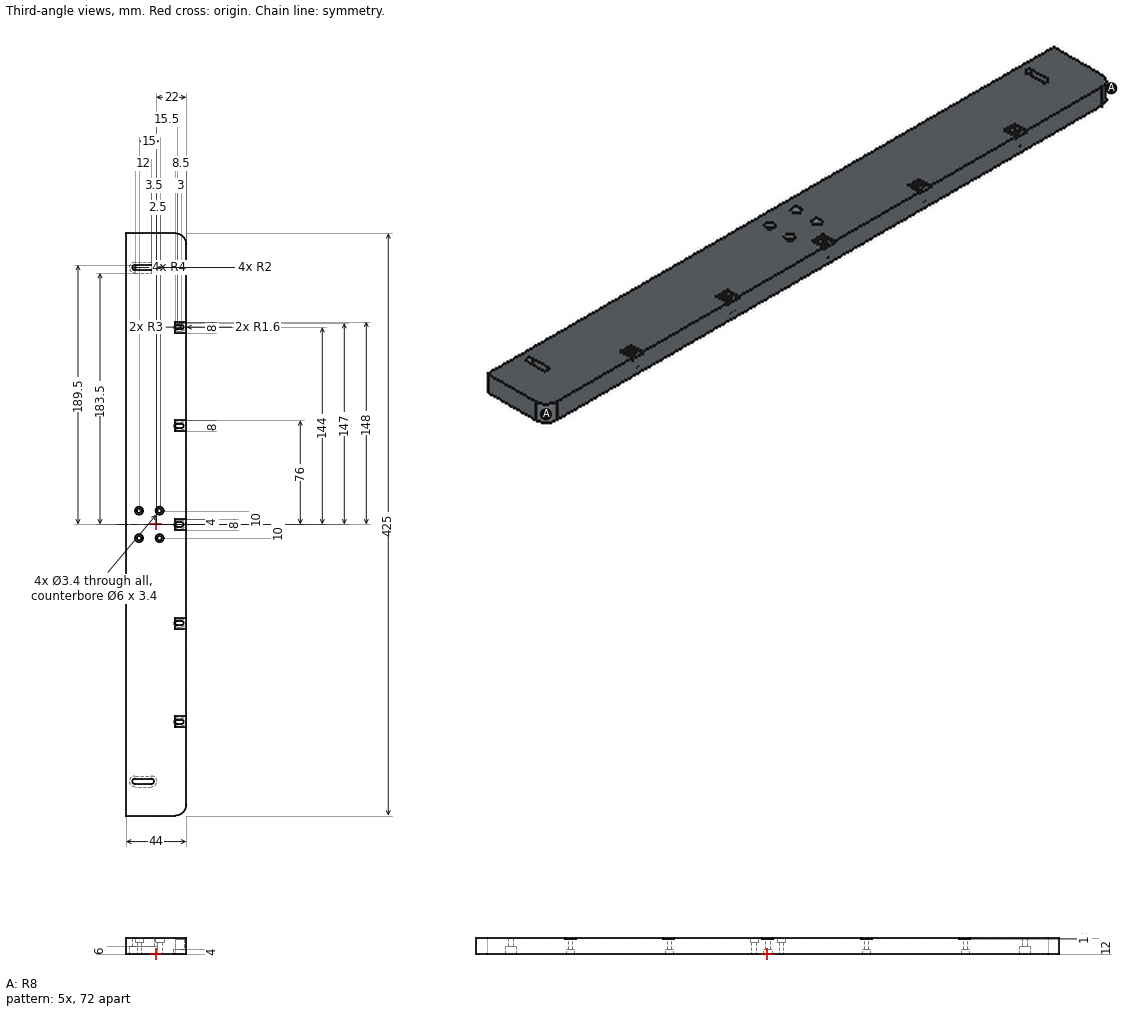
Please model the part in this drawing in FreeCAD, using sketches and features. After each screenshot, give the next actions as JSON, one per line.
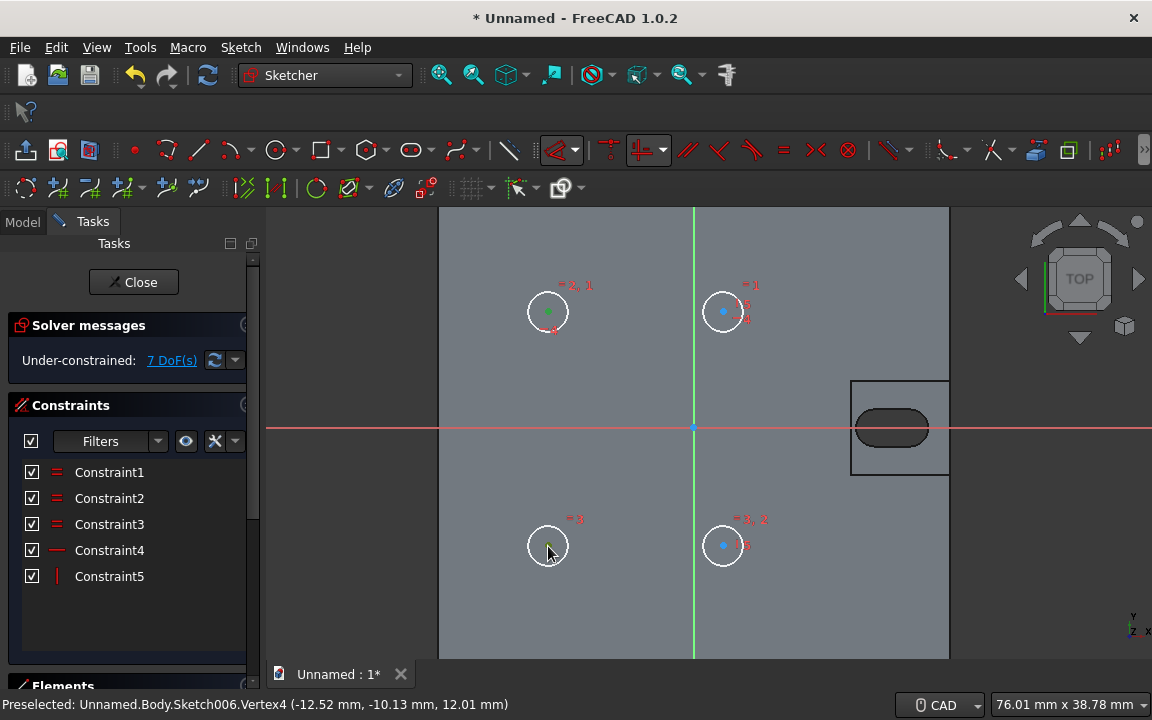
{"action": "key", "text": "v"}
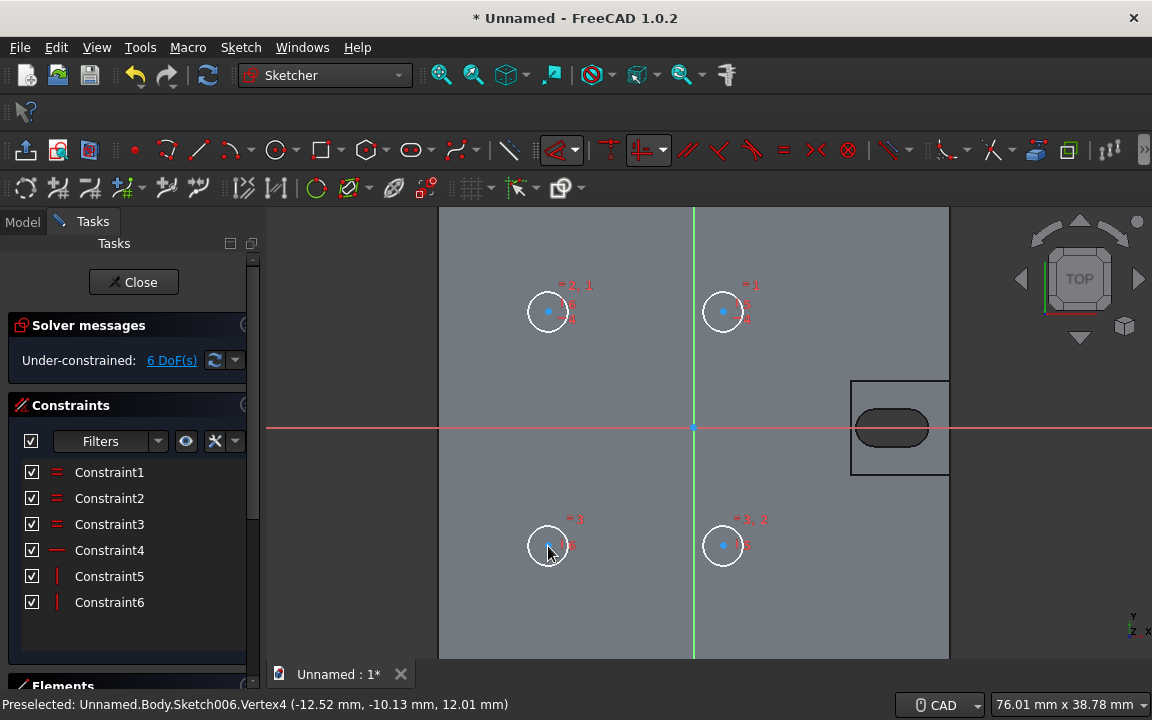
{"action": "left_click", "coordinate": [723, 546]}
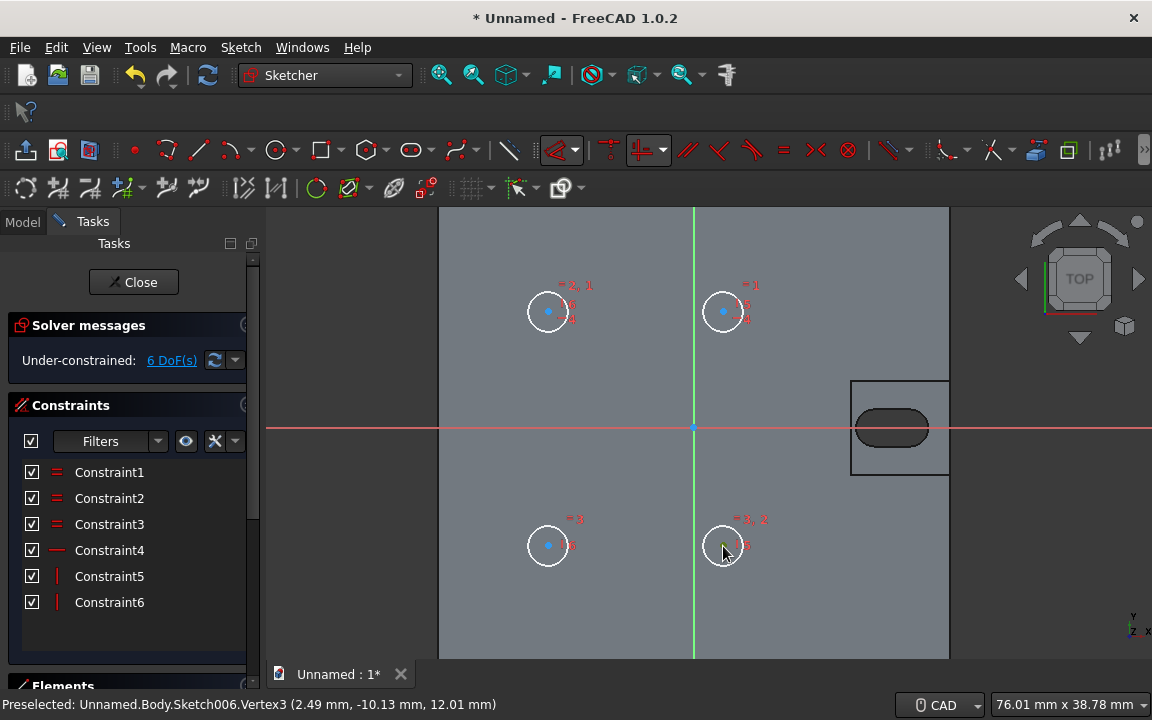
{"action": "left_click", "coordinate": [548, 546]}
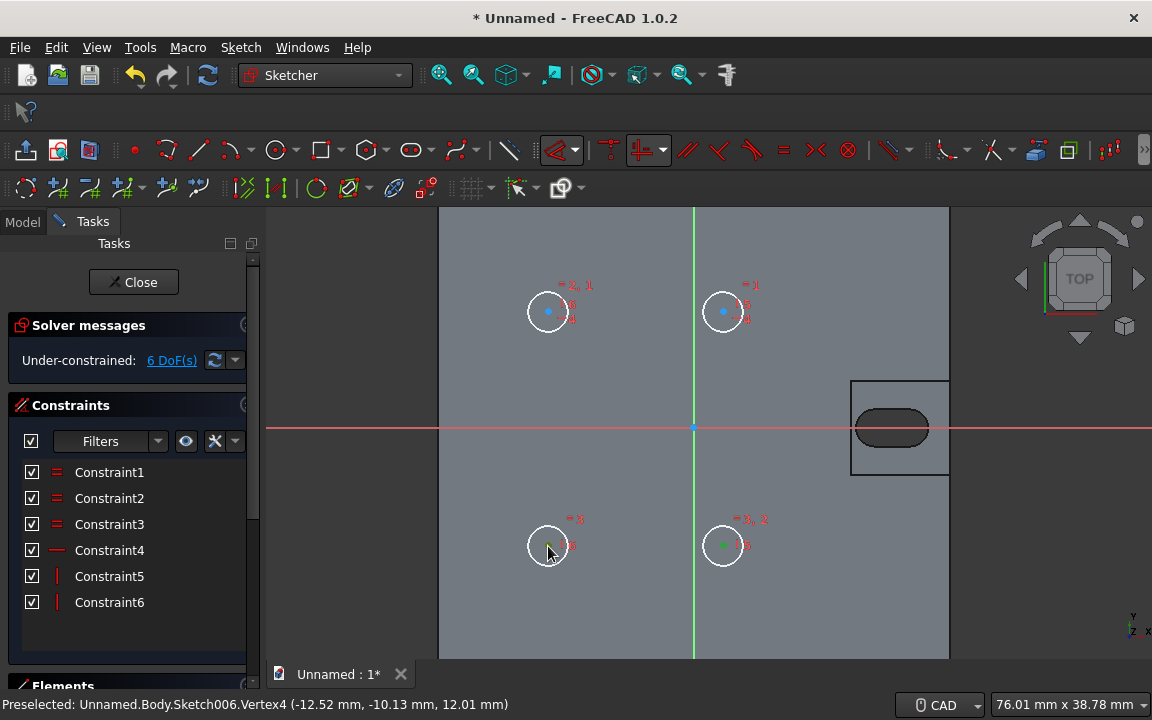
{"action": "key", "text": "h"}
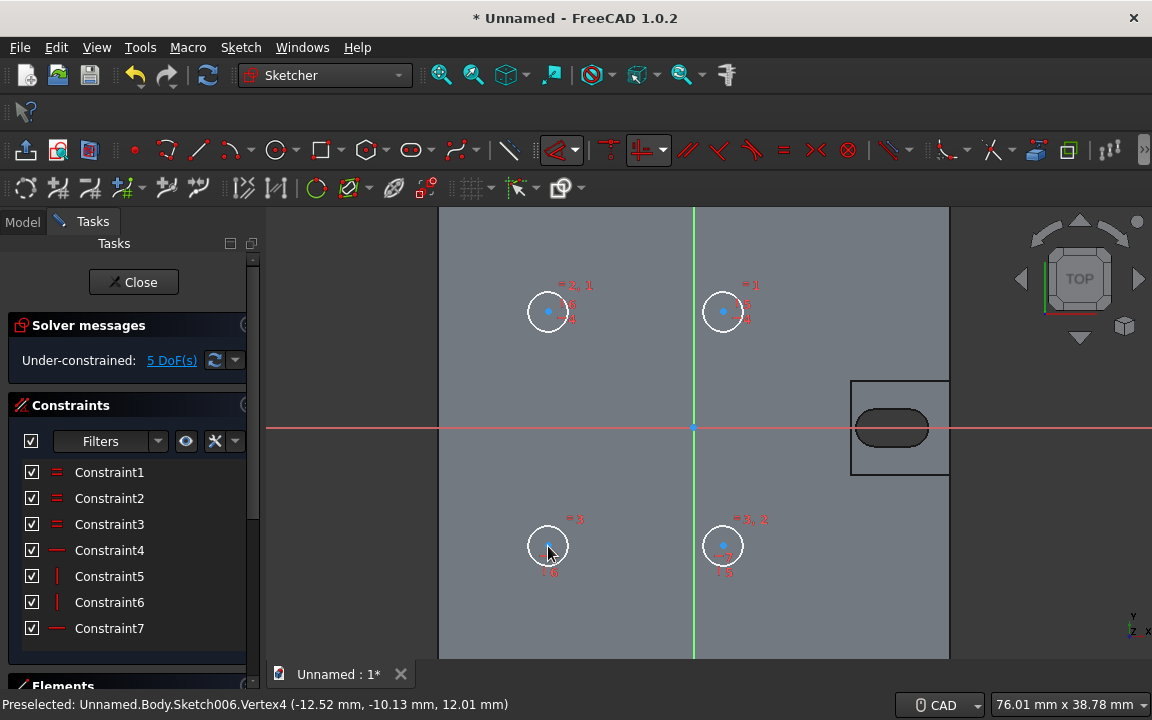
{"action": "left_click", "coordinate": [709, 298]}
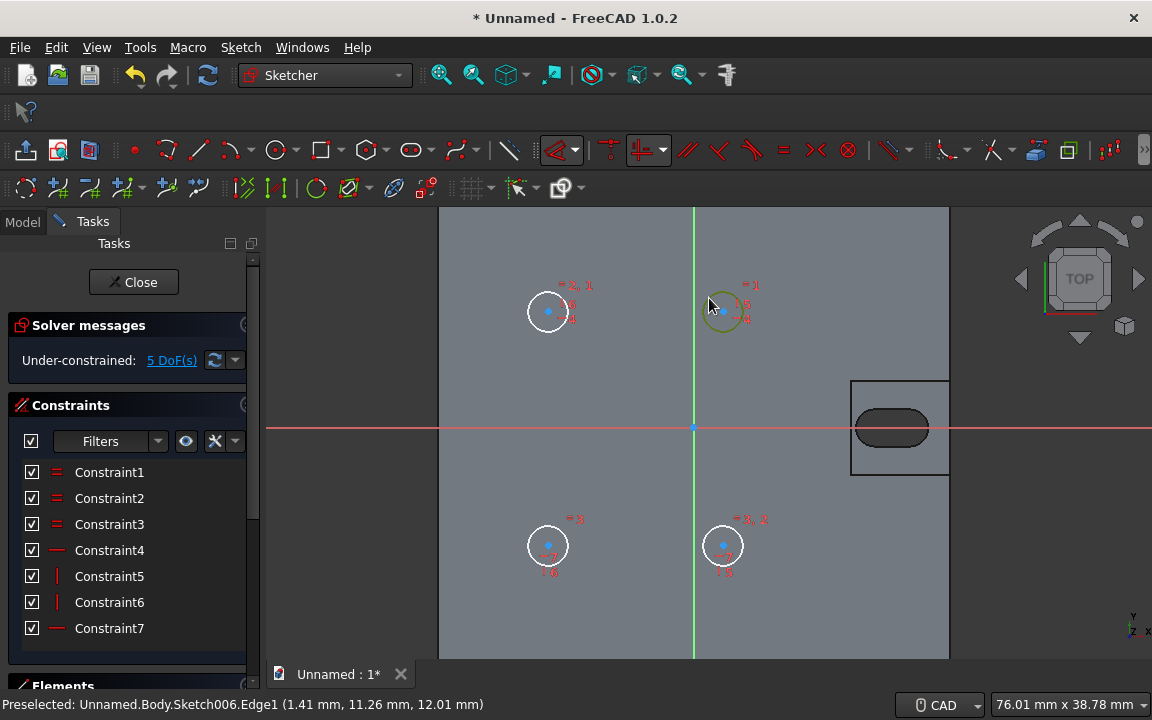
{"action": "key", "text": "k o"}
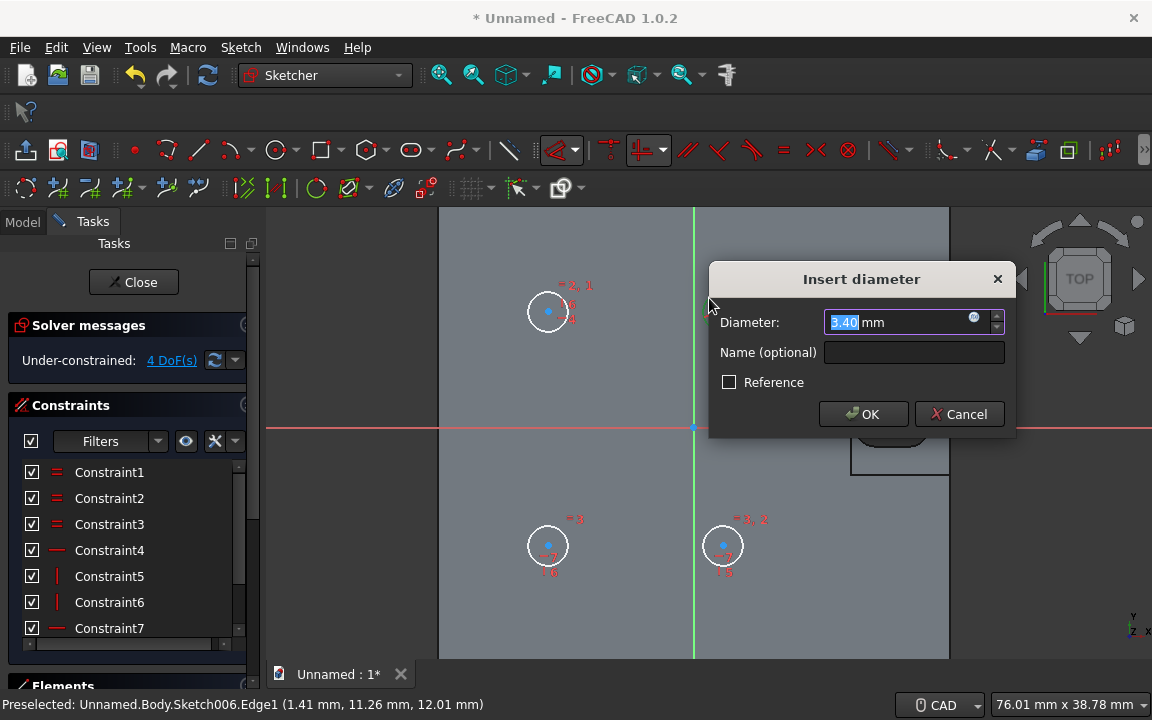
{"action": "type", "text": "3.4"}
{"action": "key", "text": "Return"}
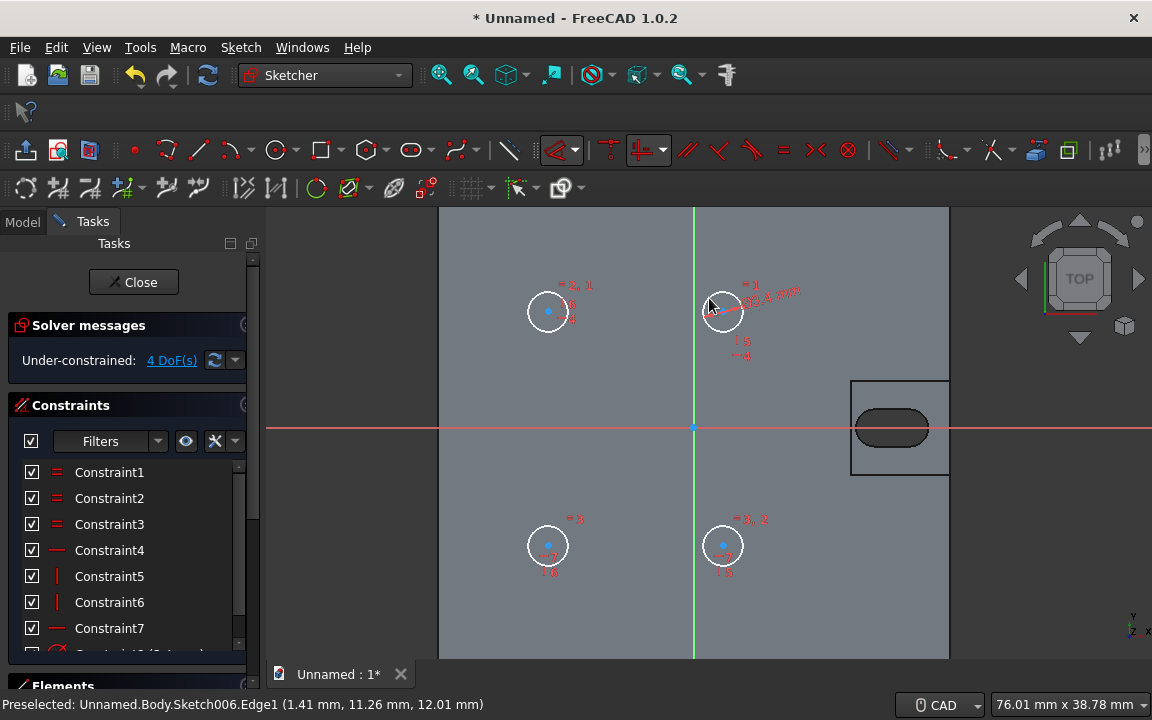
{"action": "left_click", "coordinate": [723, 312]}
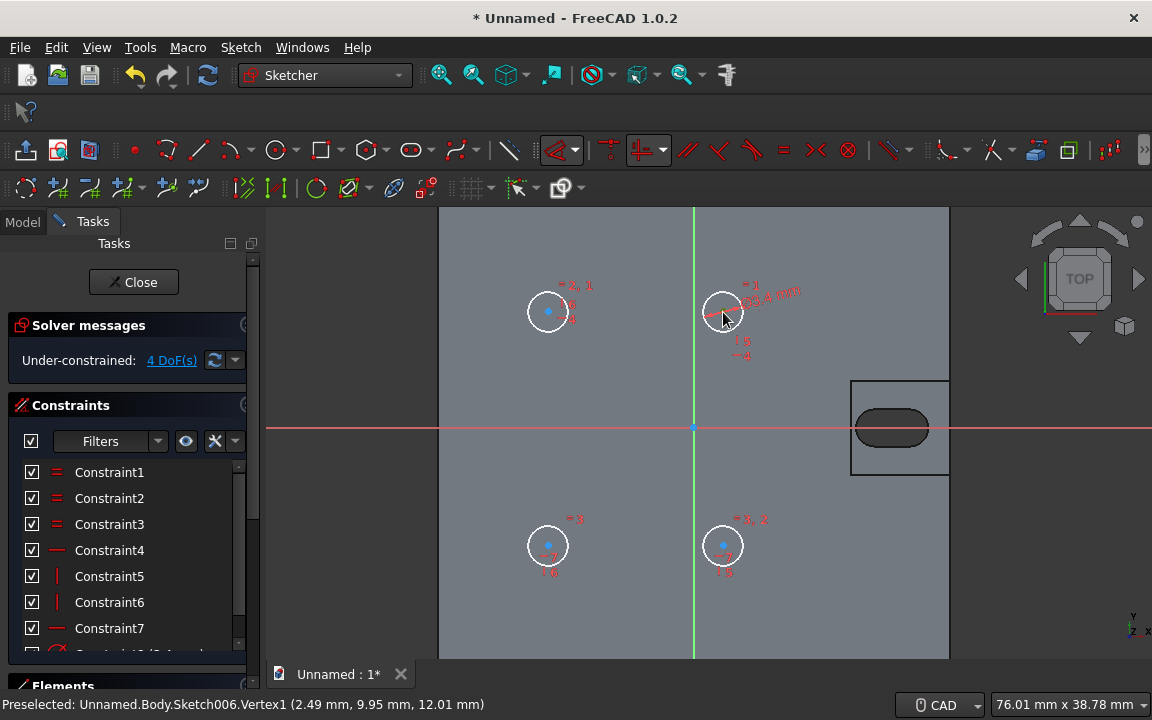
{"action": "key", "text": "i"}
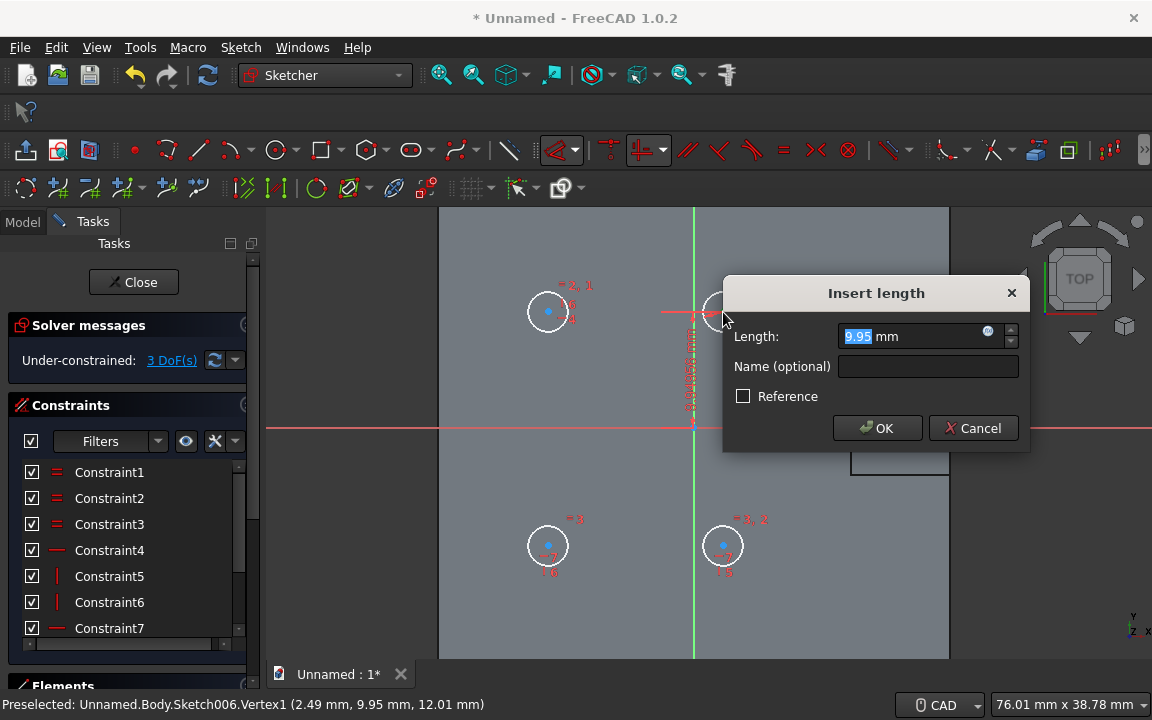
{"action": "type", "text": "10"}
{"action": "key", "text": "Return"}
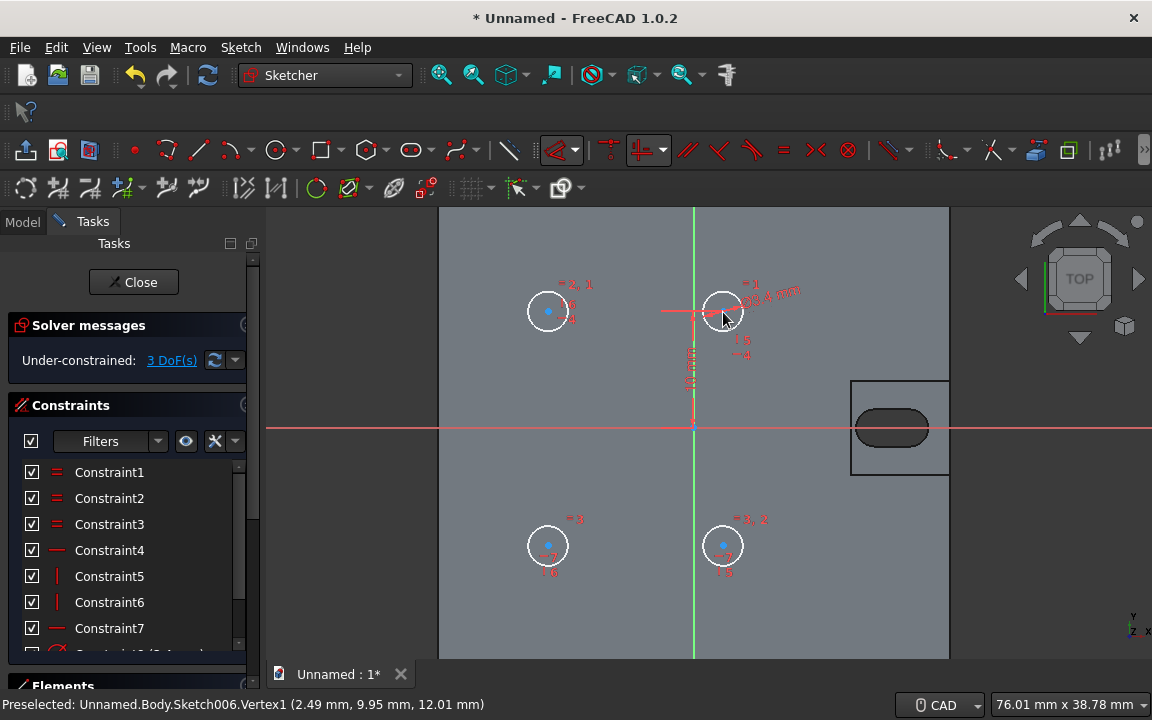
{"action": "left_click", "coordinate": [723, 546]}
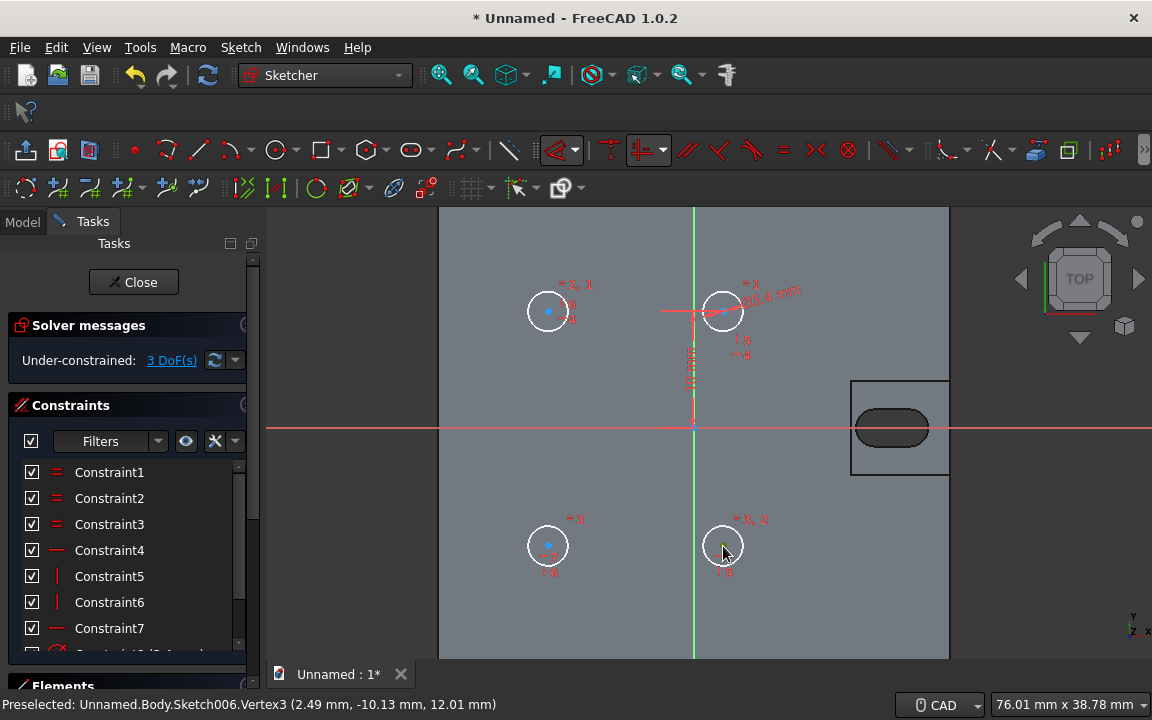
{"action": "key", "text": "i"}